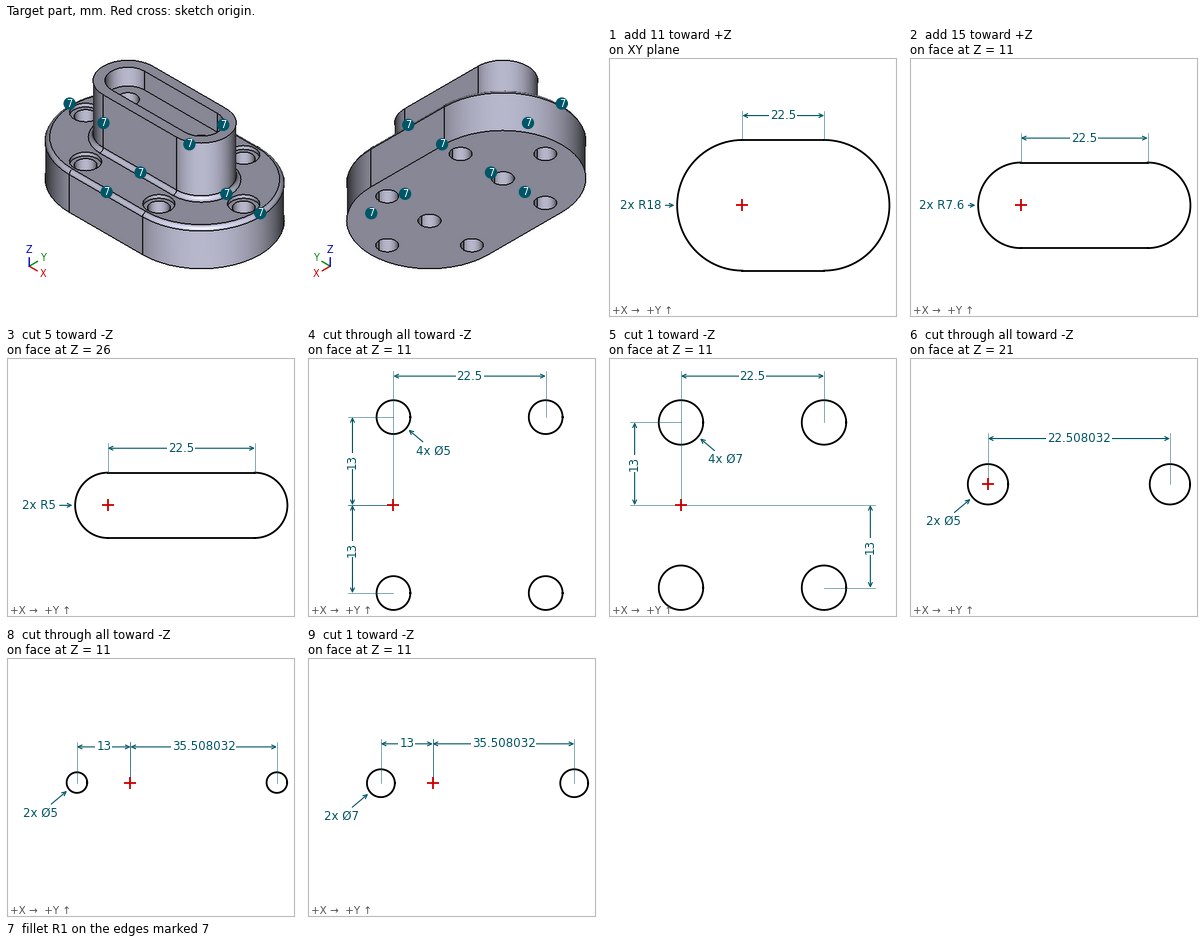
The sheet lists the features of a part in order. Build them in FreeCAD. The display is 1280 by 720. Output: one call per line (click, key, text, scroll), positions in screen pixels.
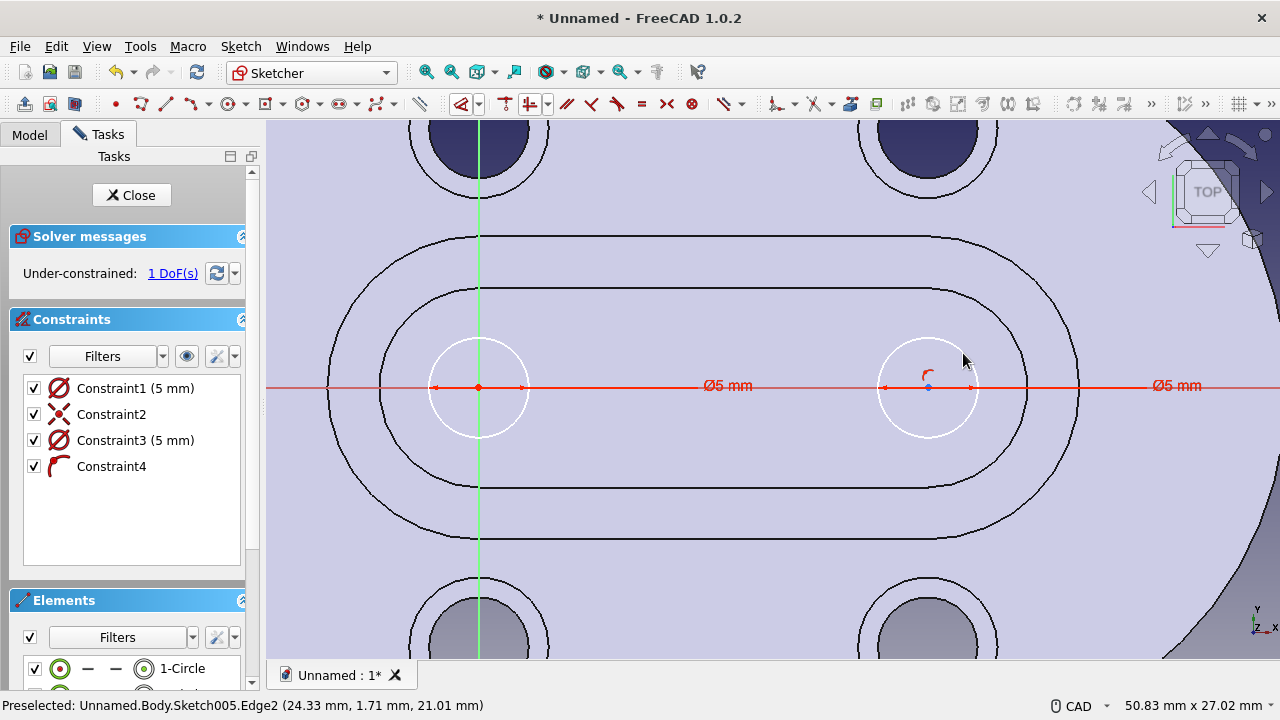
click(928, 388)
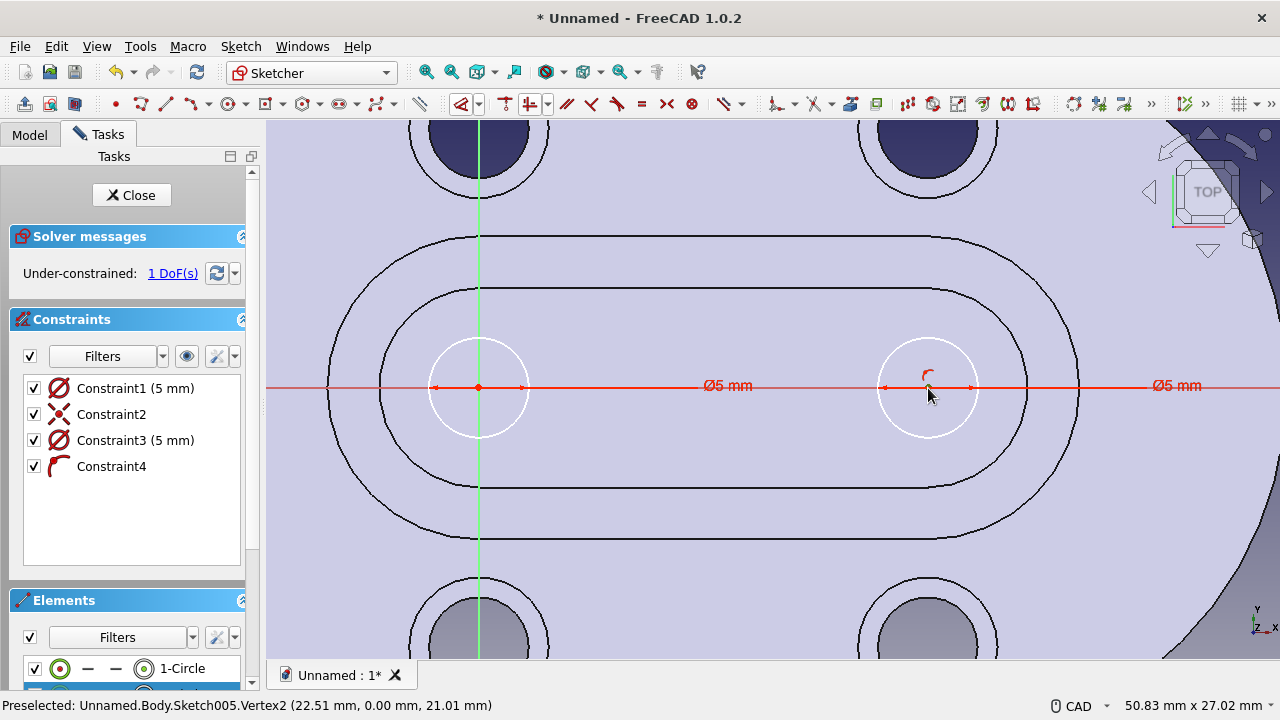
key(l)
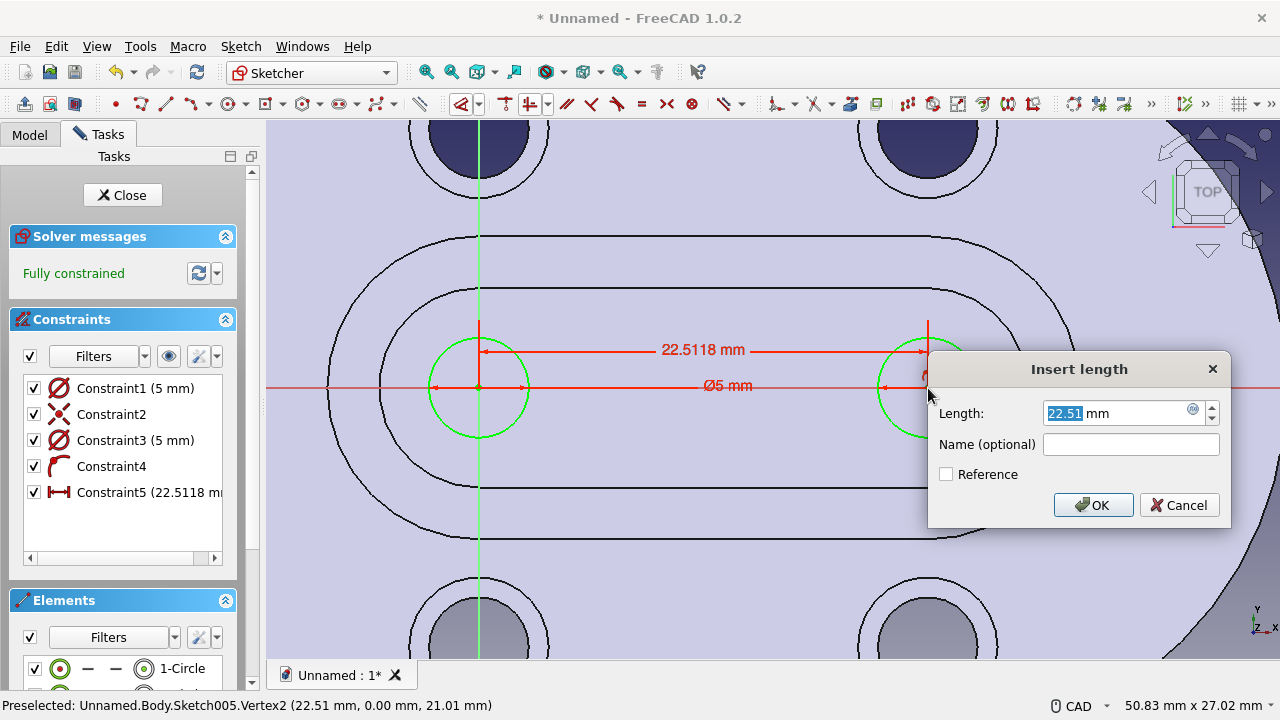
text(22.508032)
key(Return)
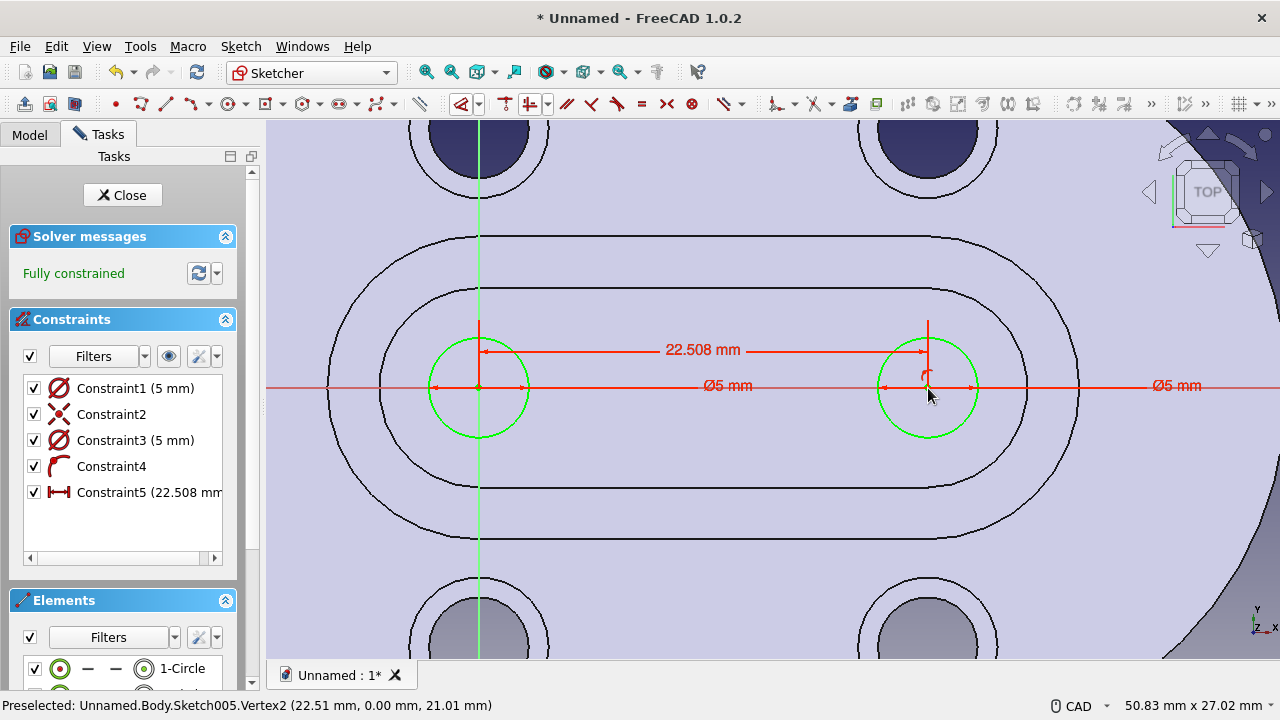
click(123, 195)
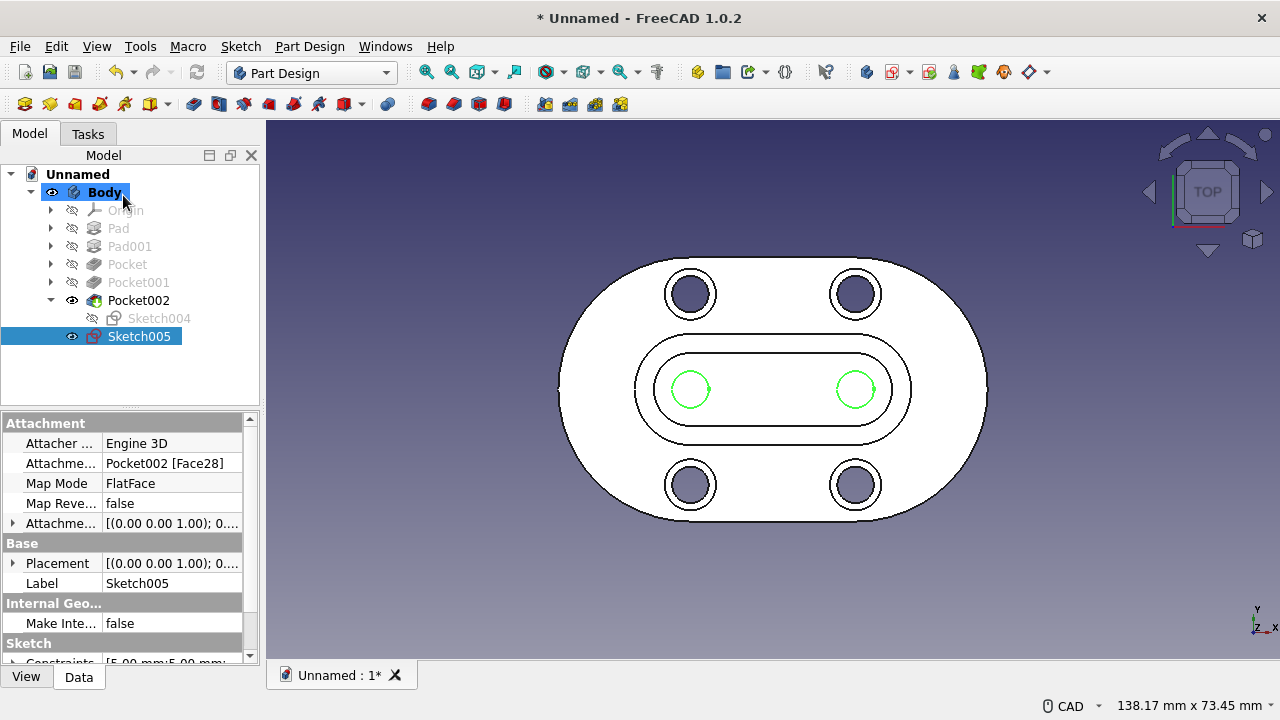
click(194, 104)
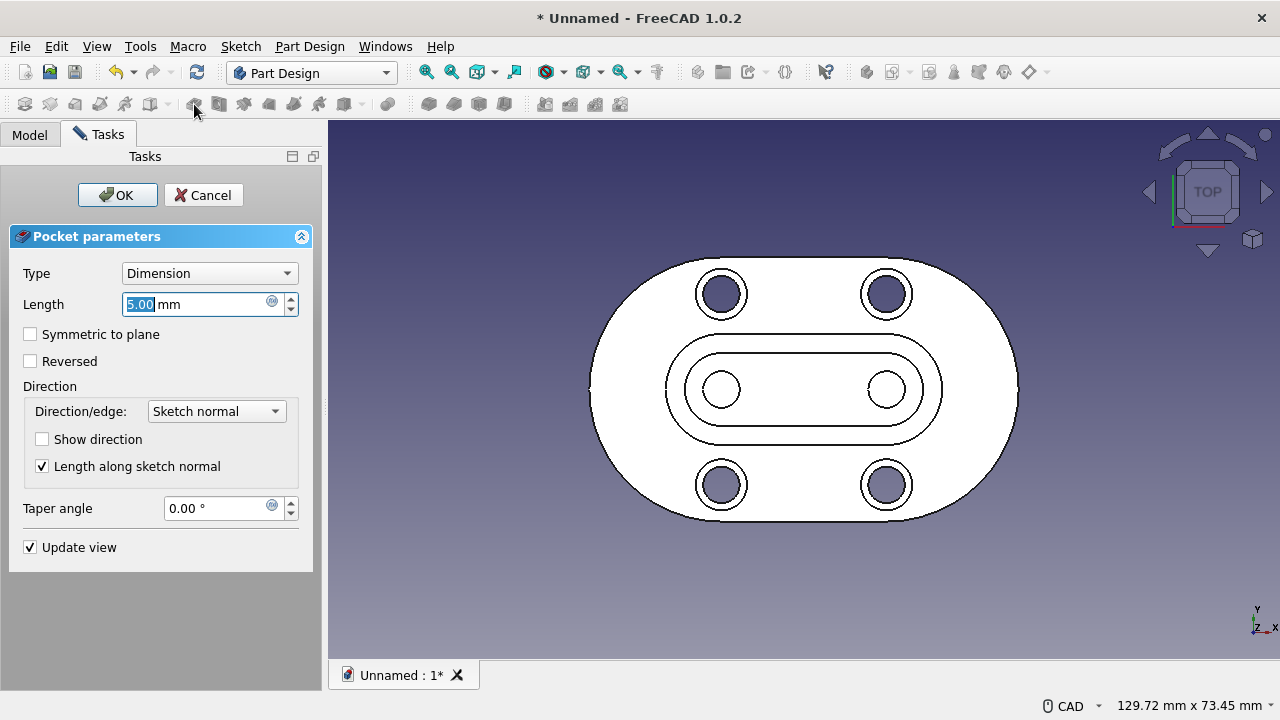
click(210, 274)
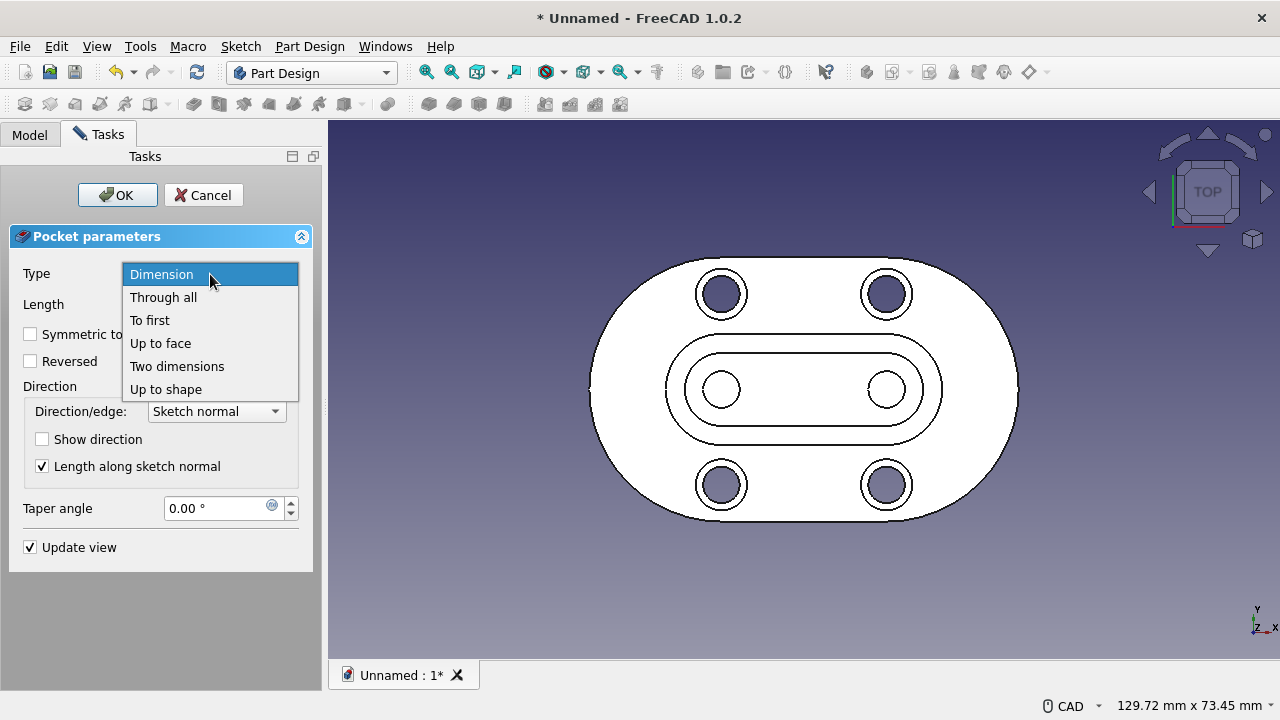
click(208, 298)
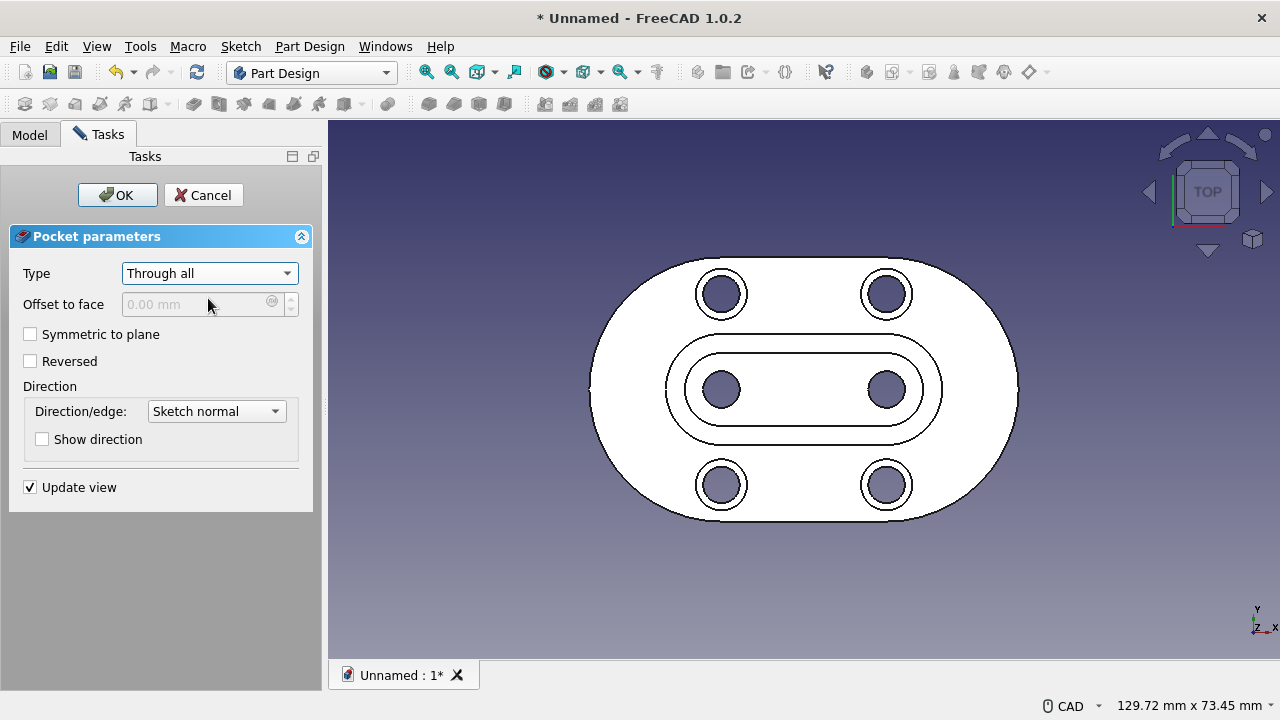
click(118, 195)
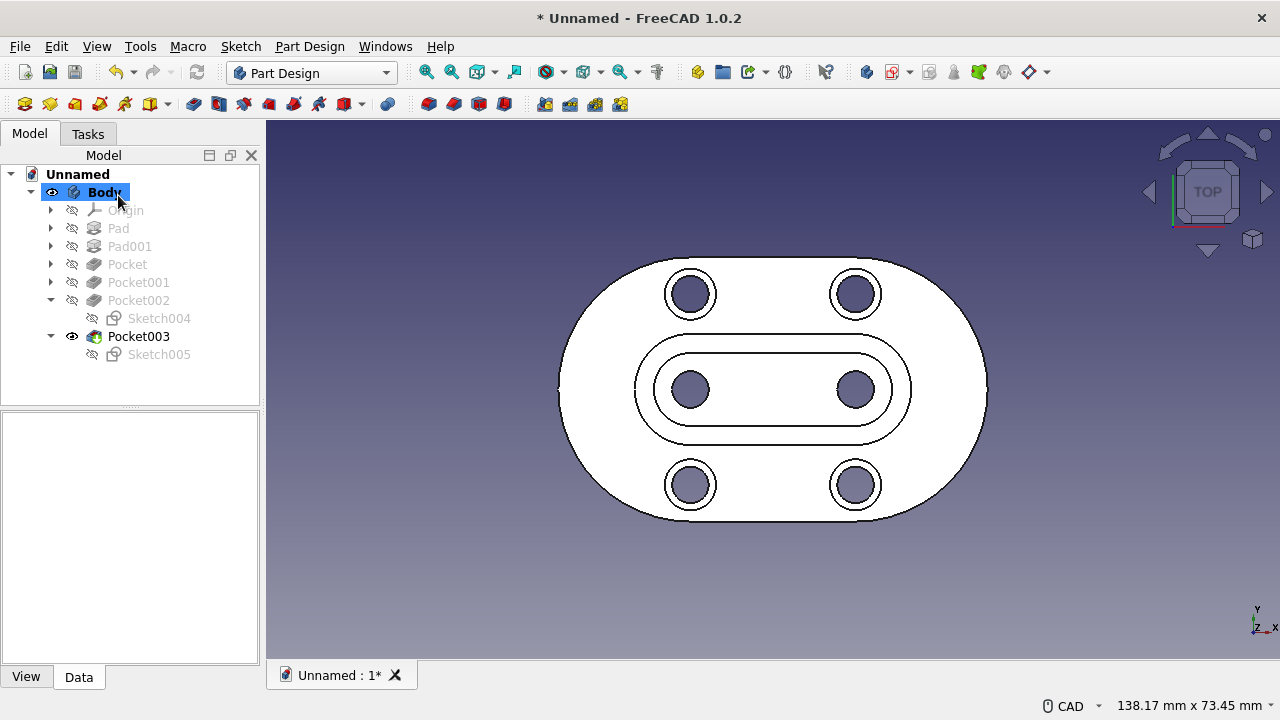
click(988, 389)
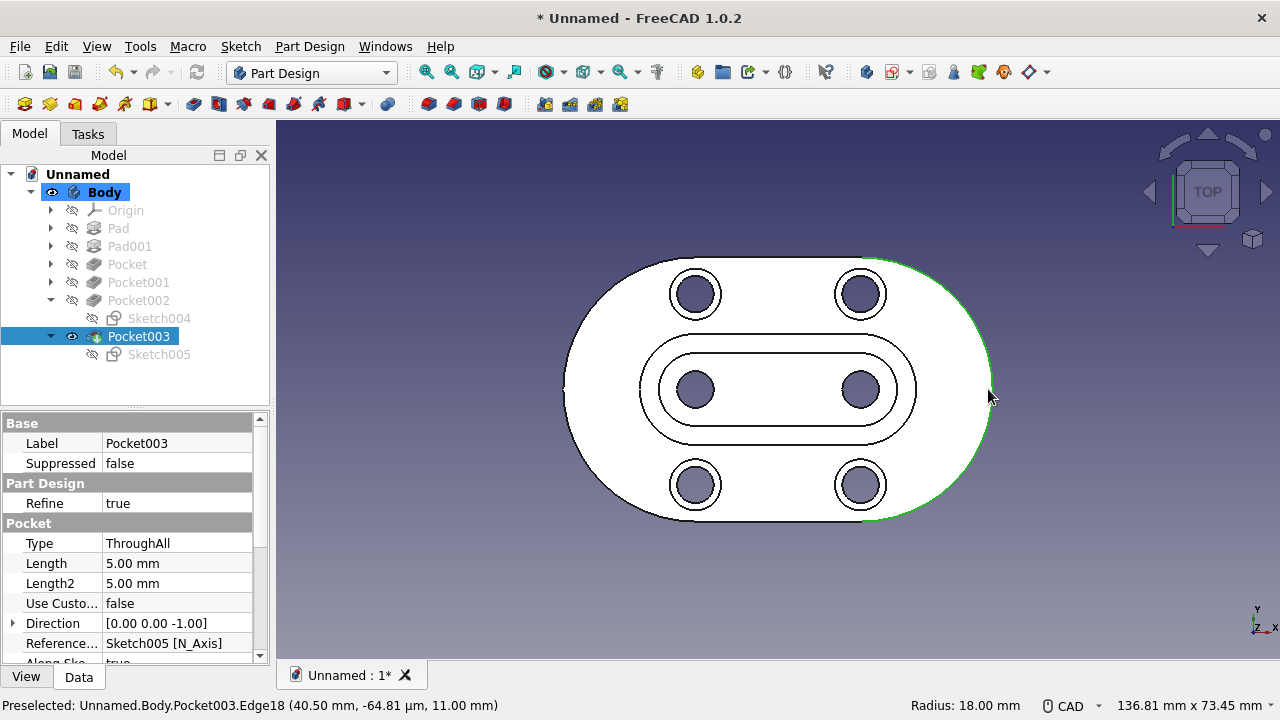
click(778, 256, ctrl)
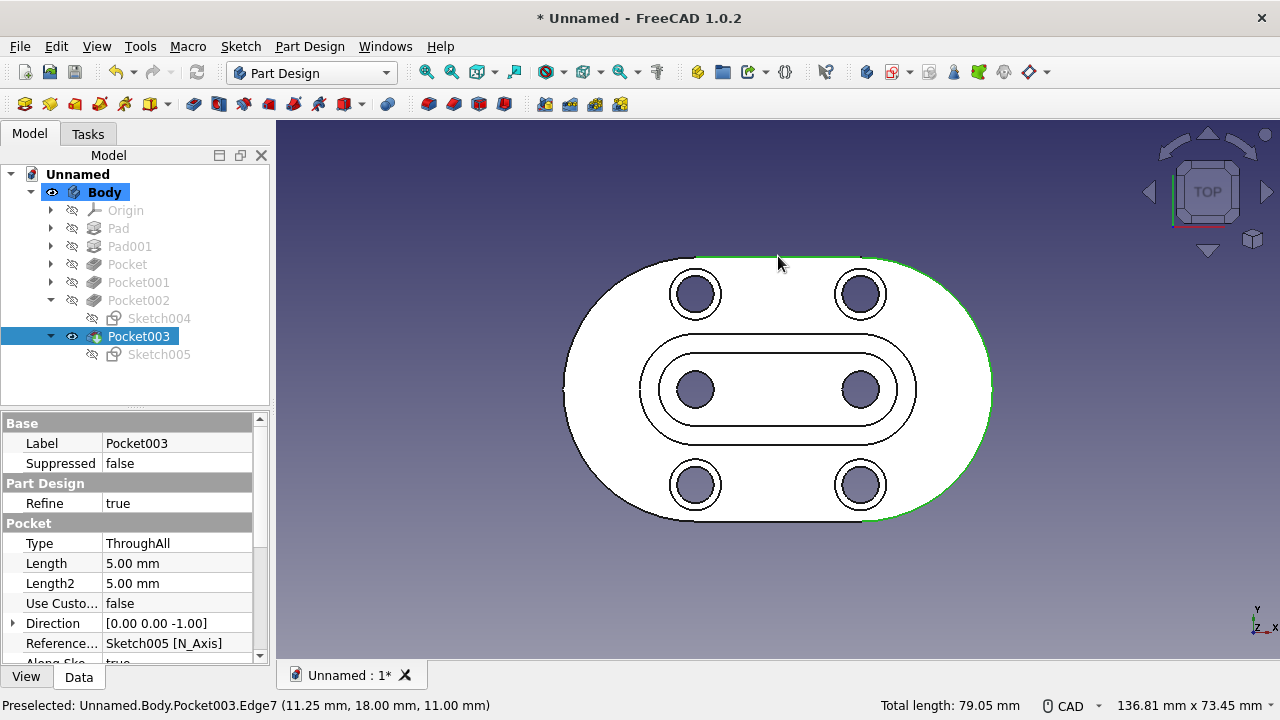
click(563, 389, ctrl)